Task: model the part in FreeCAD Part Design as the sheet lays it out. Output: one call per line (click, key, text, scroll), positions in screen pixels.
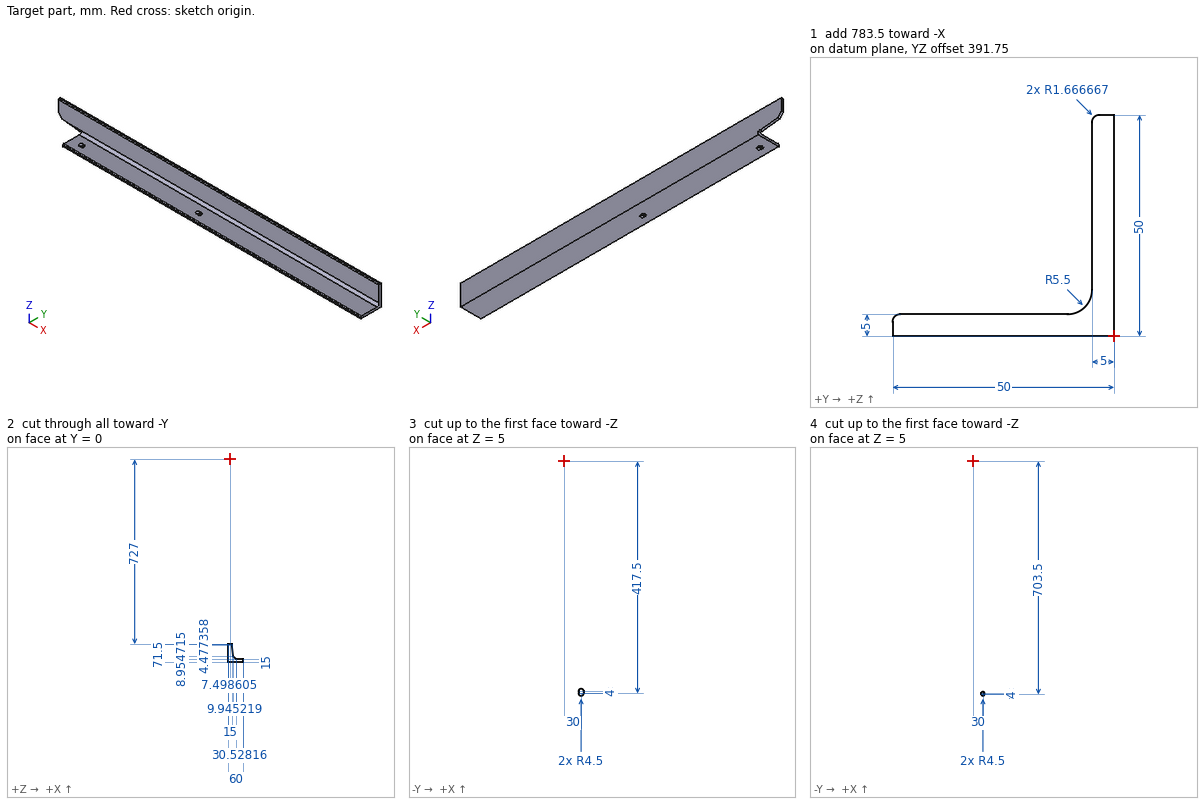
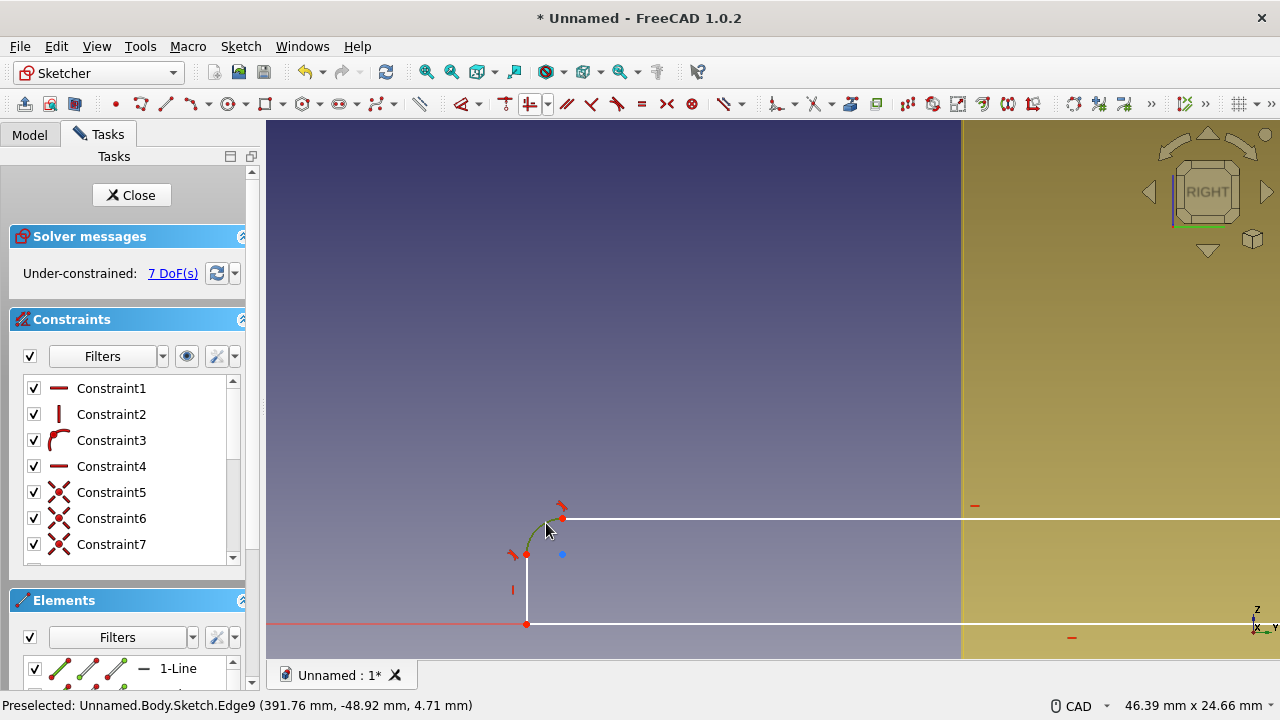
click(642, 104)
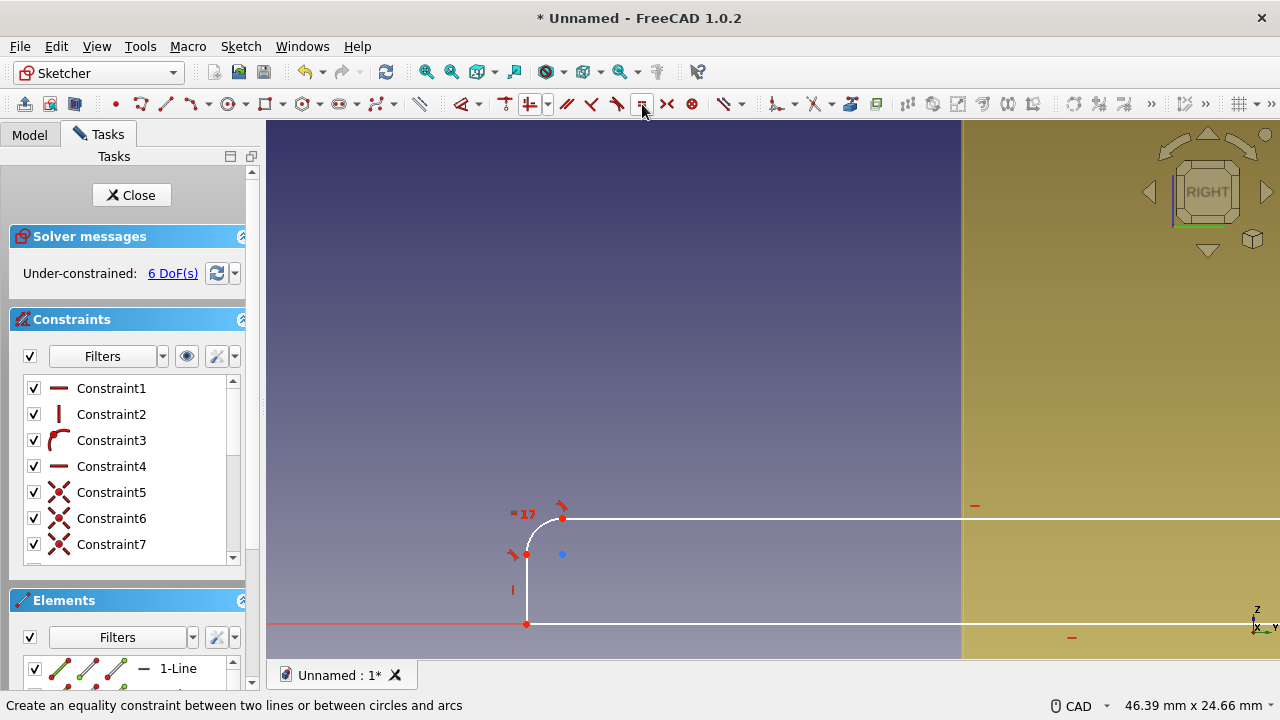
scroll(546, 524, down, 6)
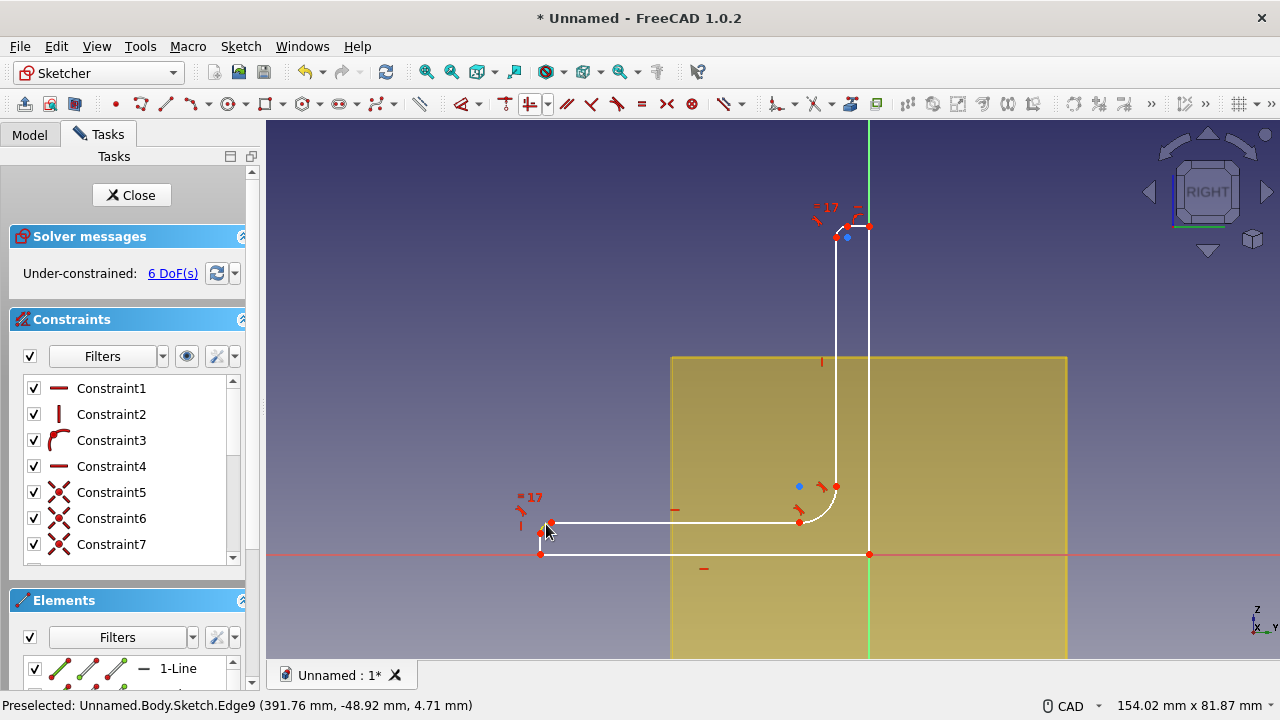
click(816, 519)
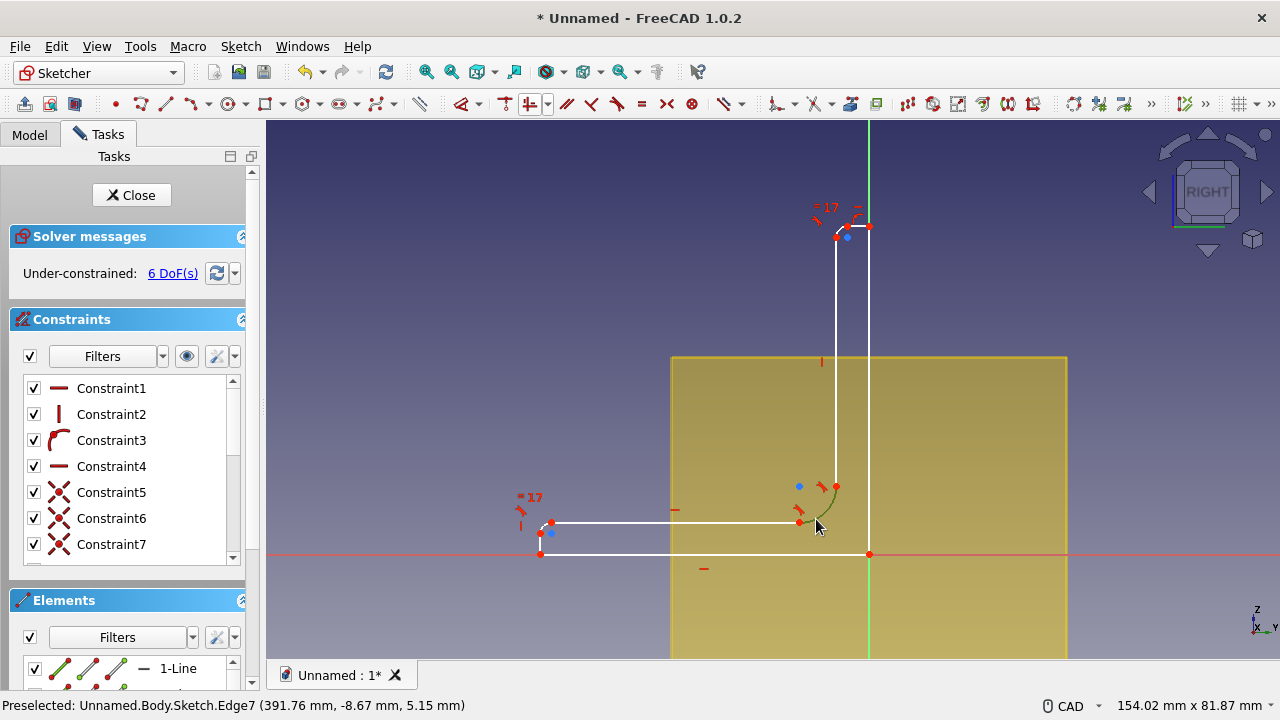
click(478, 104)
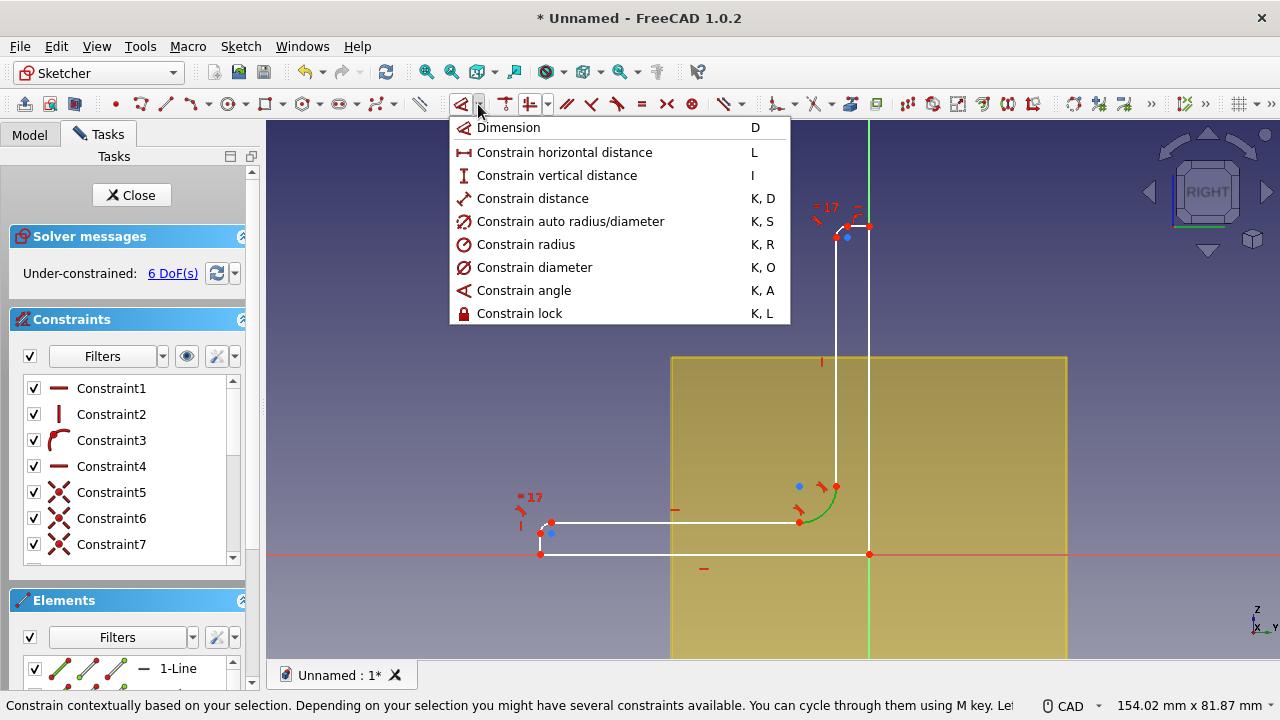
click(620, 244)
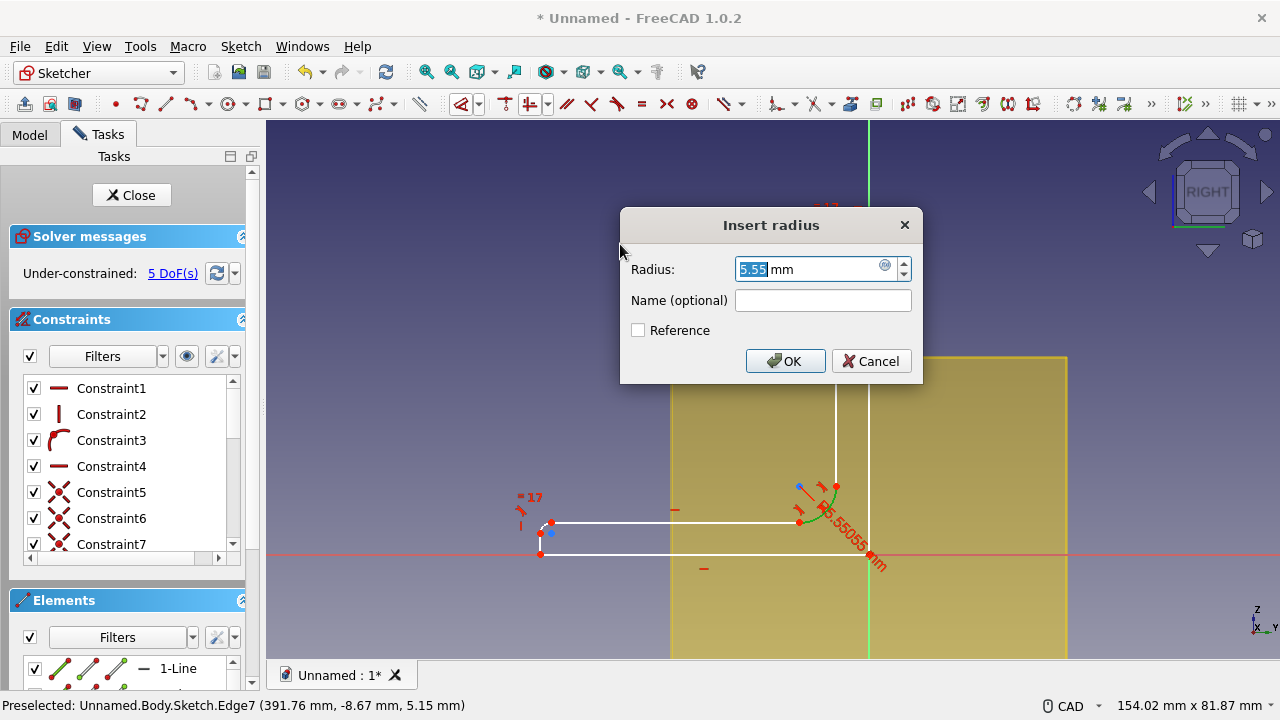
text(5.5)
key(Return)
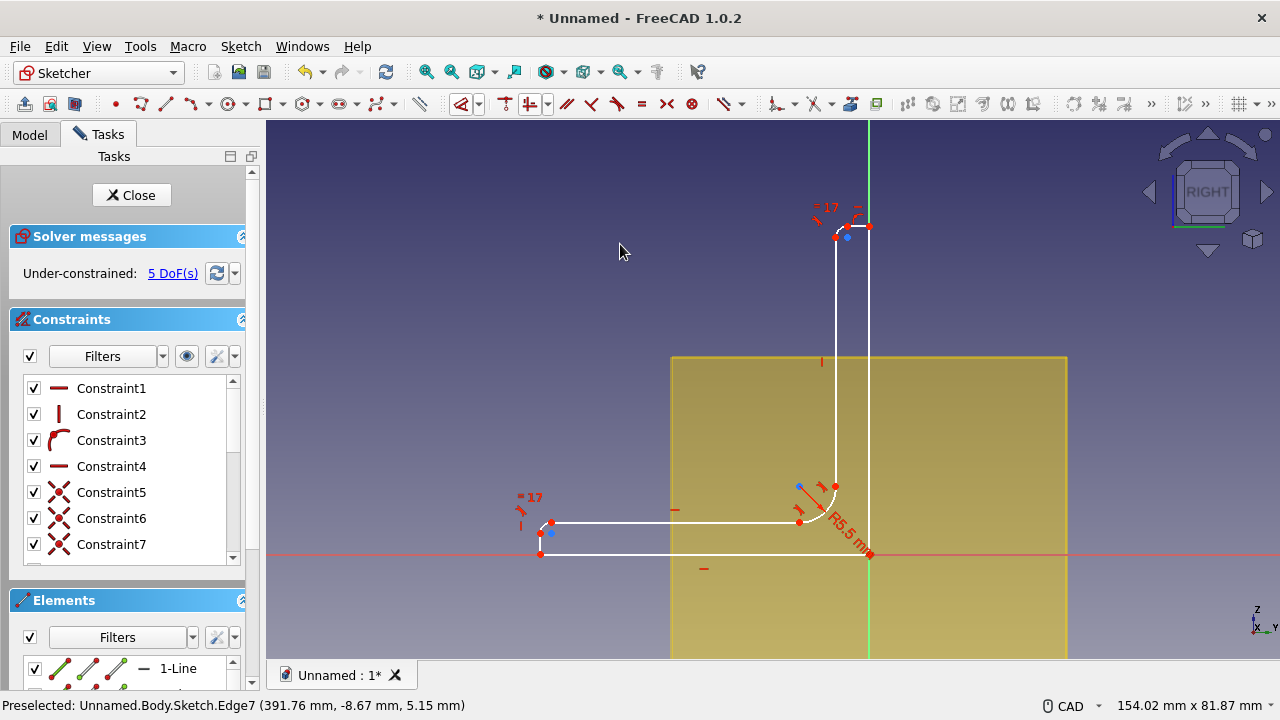
scroll(839, 230, up, 7)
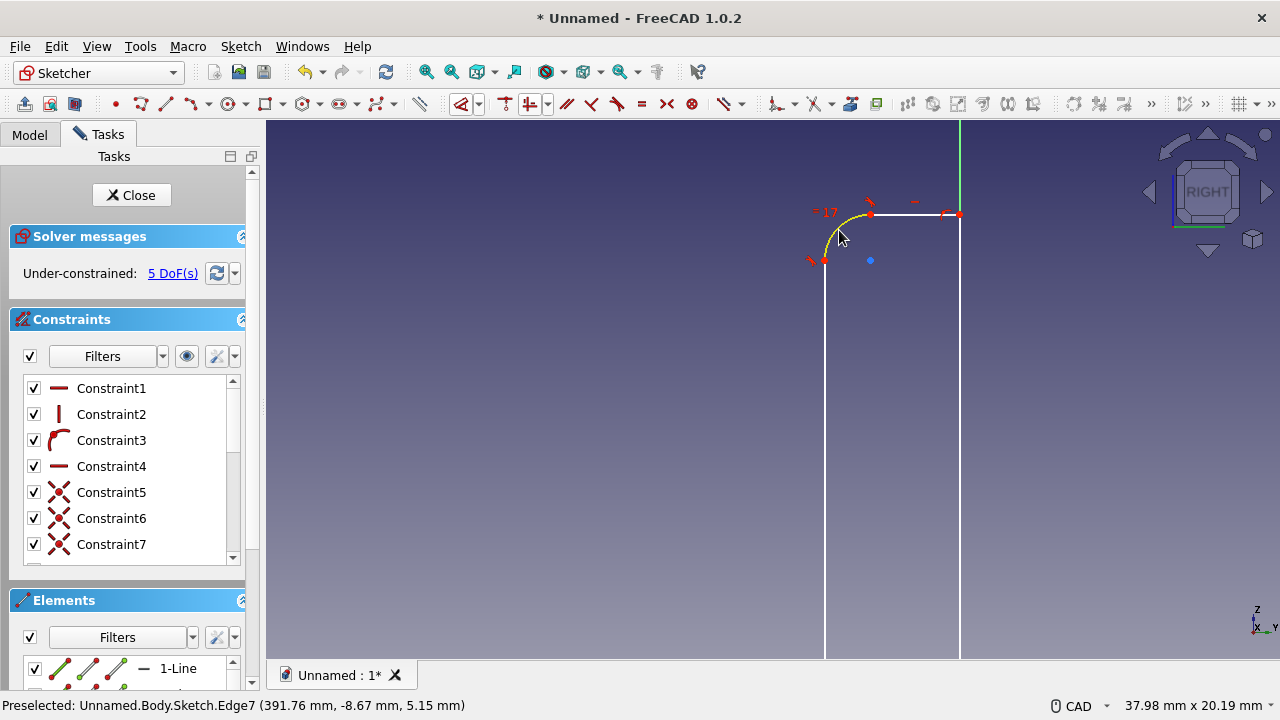
click(838, 228)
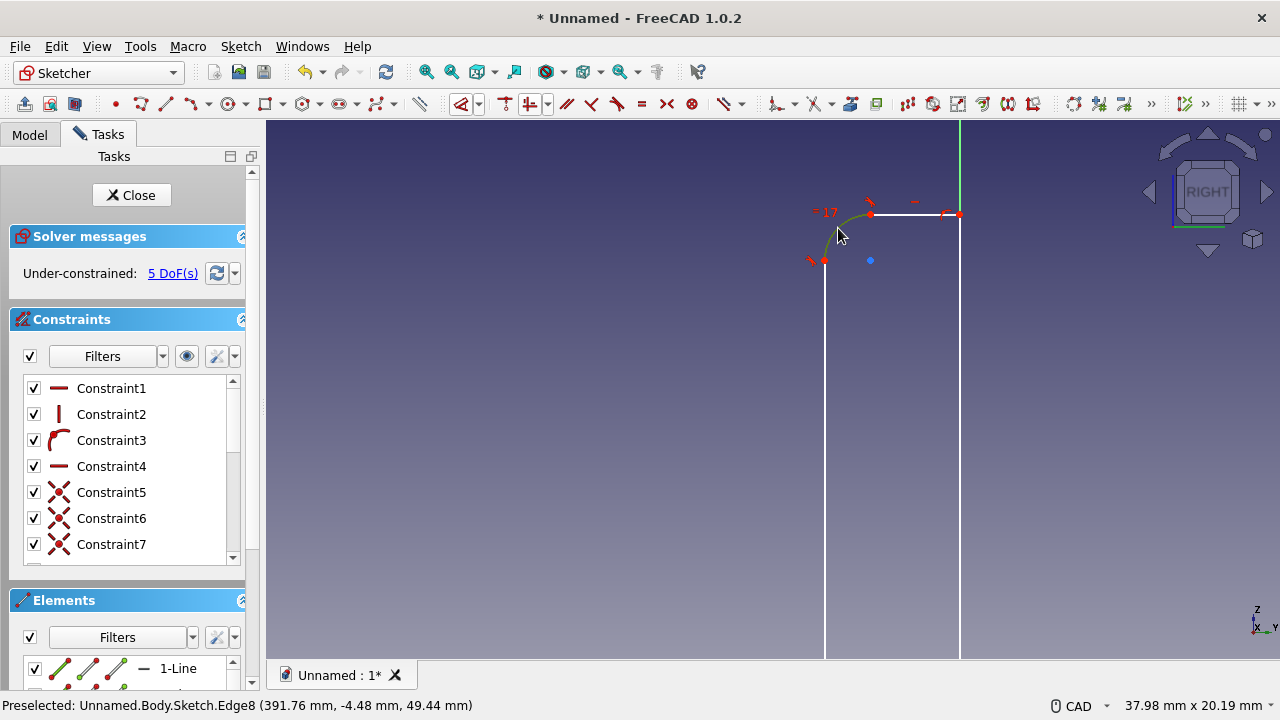
click(478, 104)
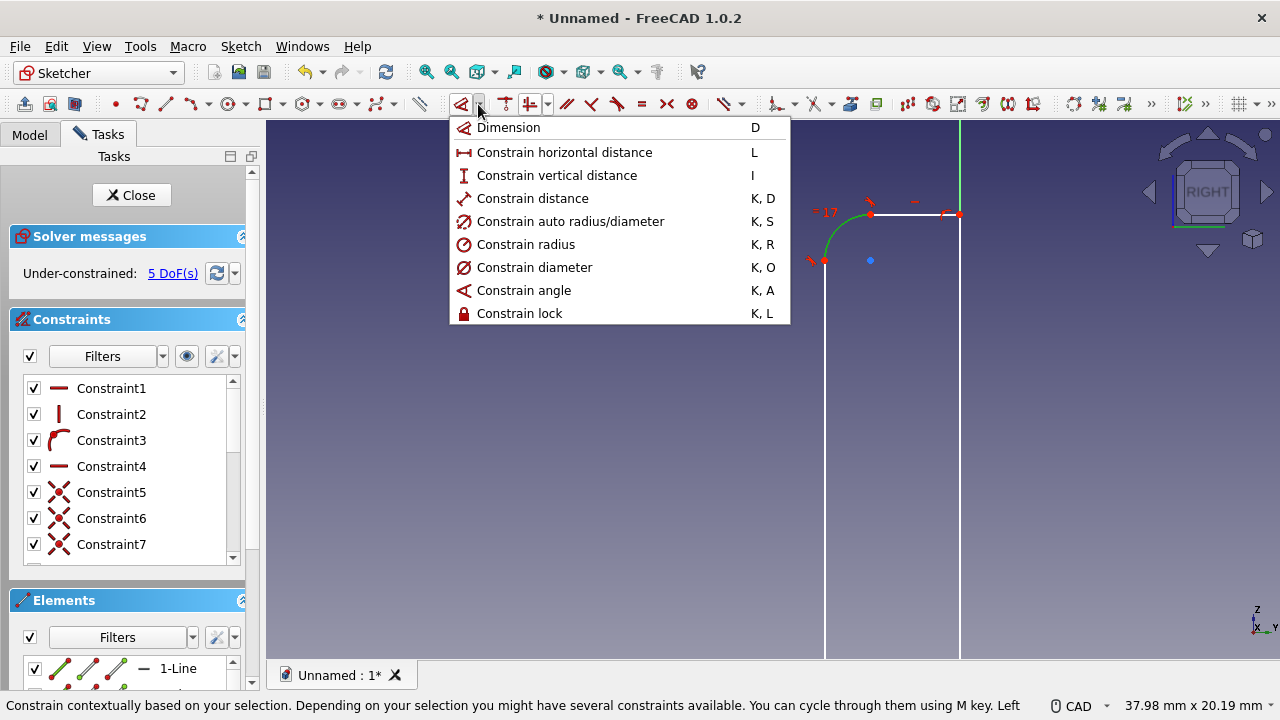
click(620, 244)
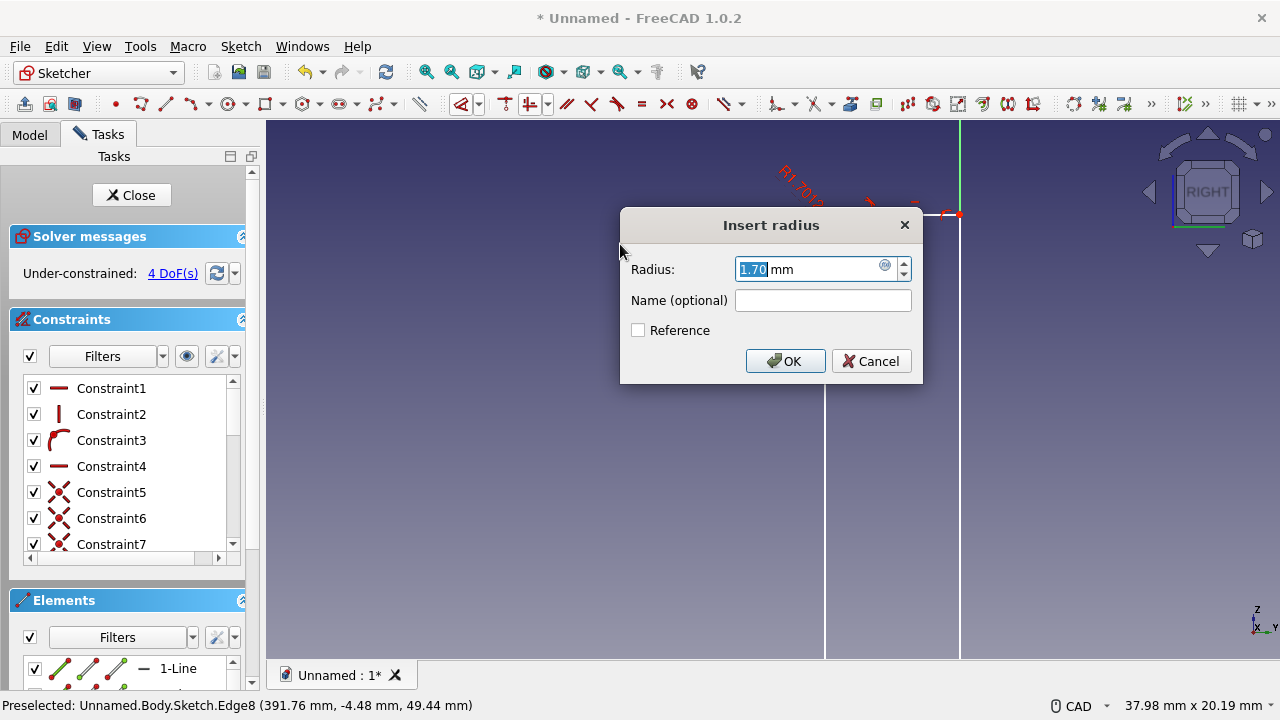
text(1.666667)
key(Return)